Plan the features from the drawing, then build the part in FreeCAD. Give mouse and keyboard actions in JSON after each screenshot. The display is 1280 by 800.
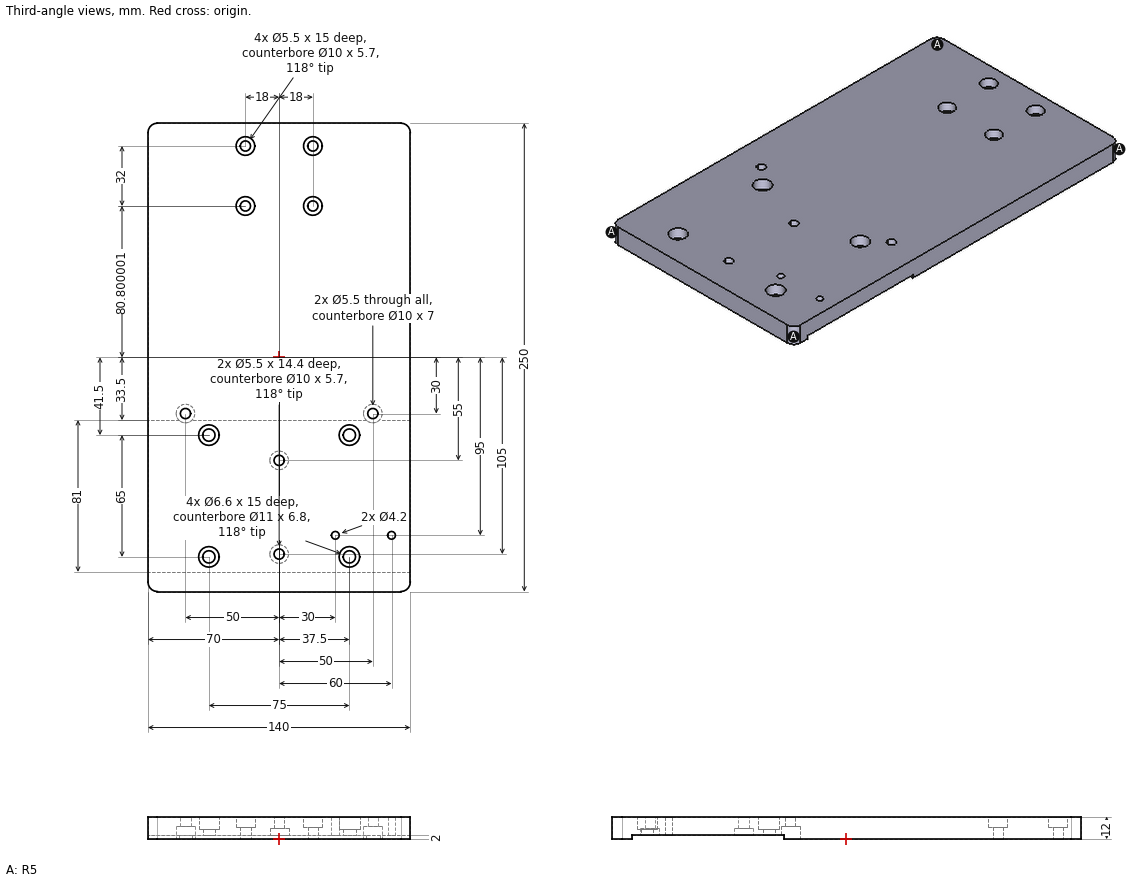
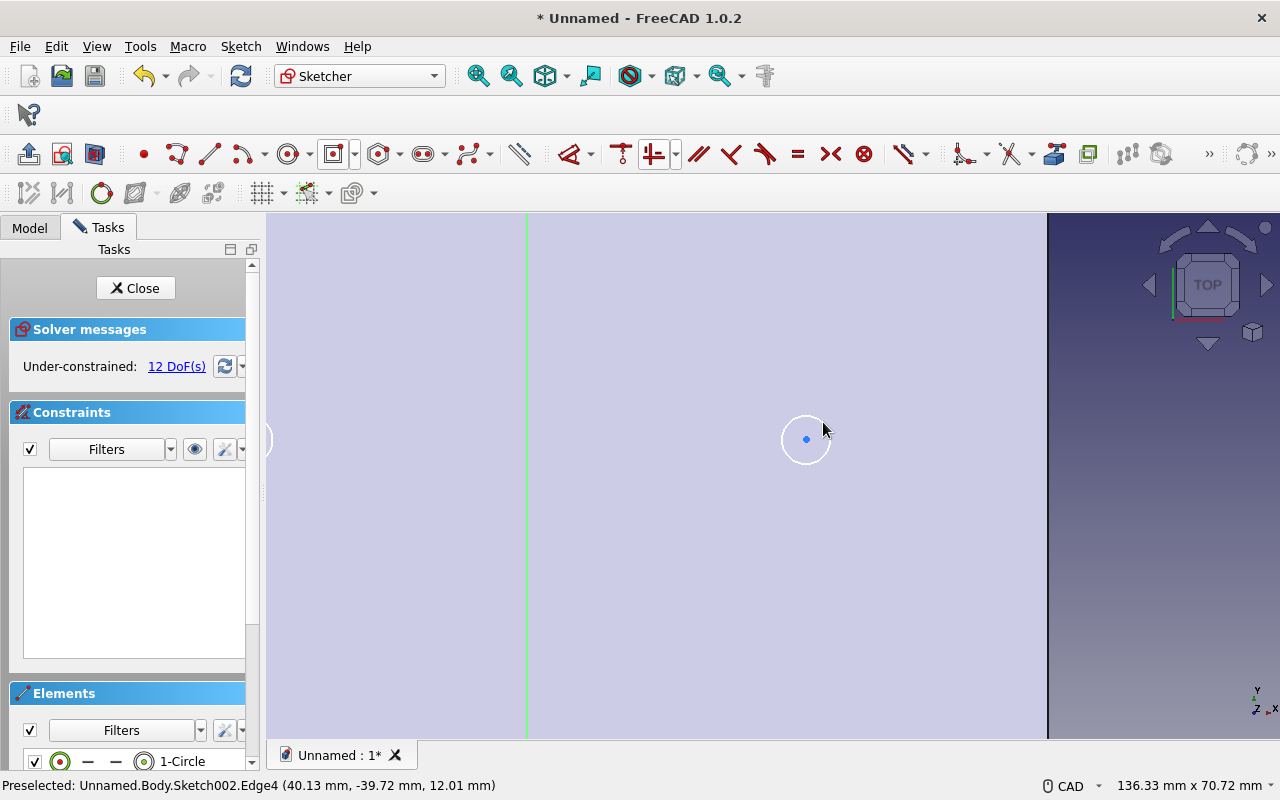
{"action": "scroll", "coordinate": [808, 439], "scroll_direction": "down", "scroll_amount": 5}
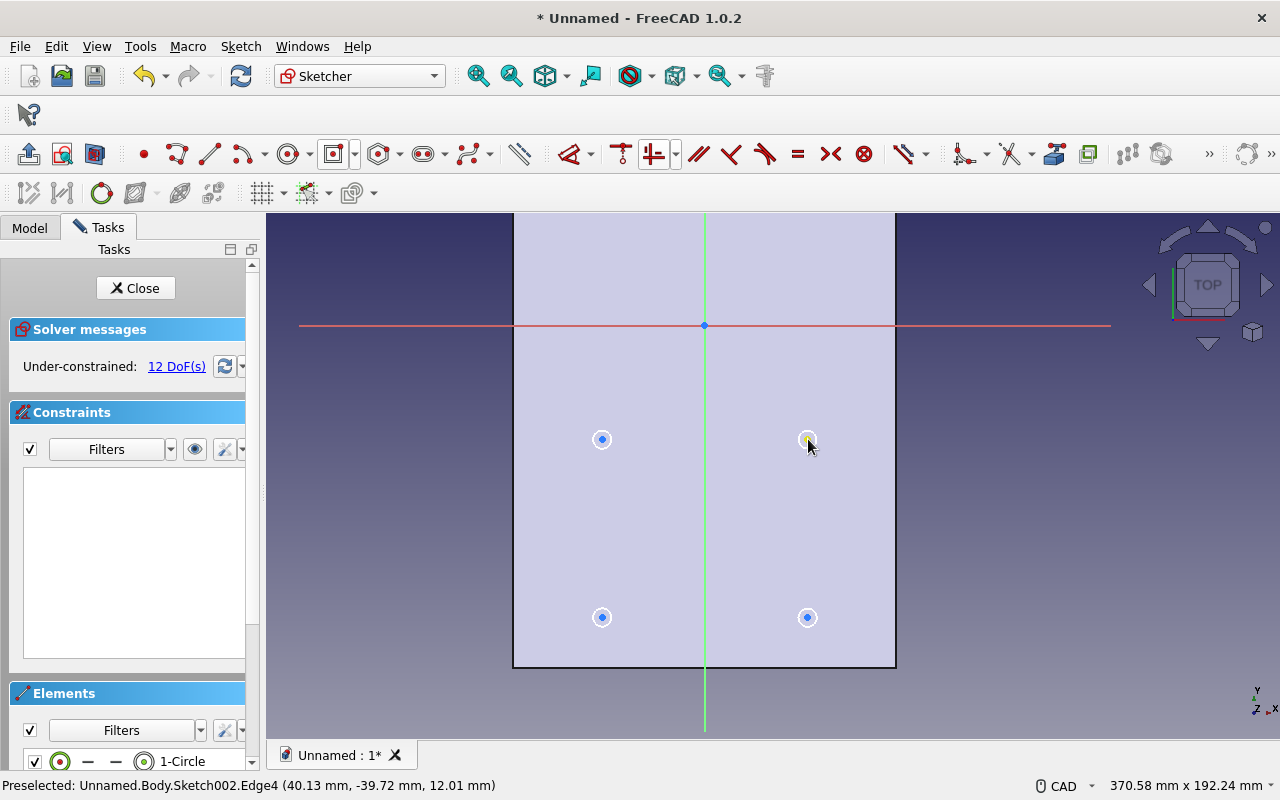
{"action": "scroll", "coordinate": [814, 611], "scroll_direction": "up", "scroll_amount": 3}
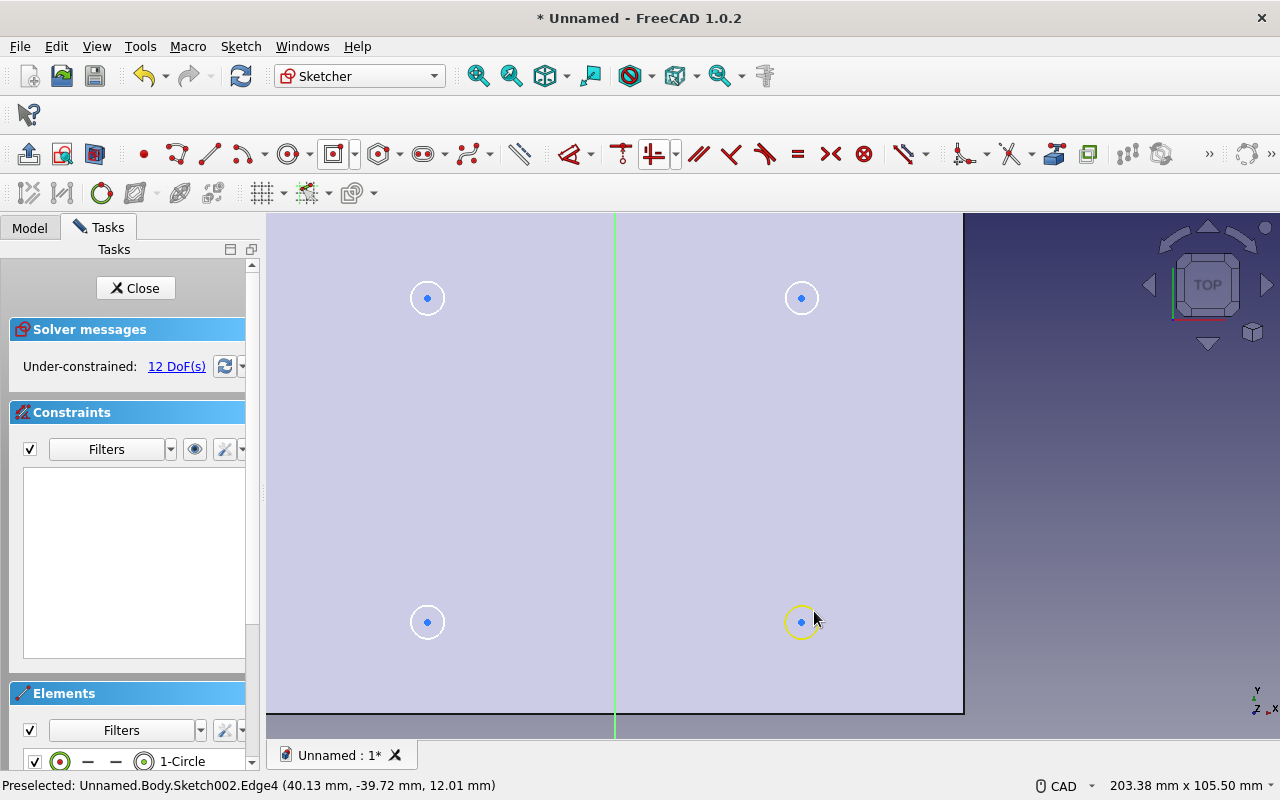
{"action": "left_click", "coordinate": [814, 611]}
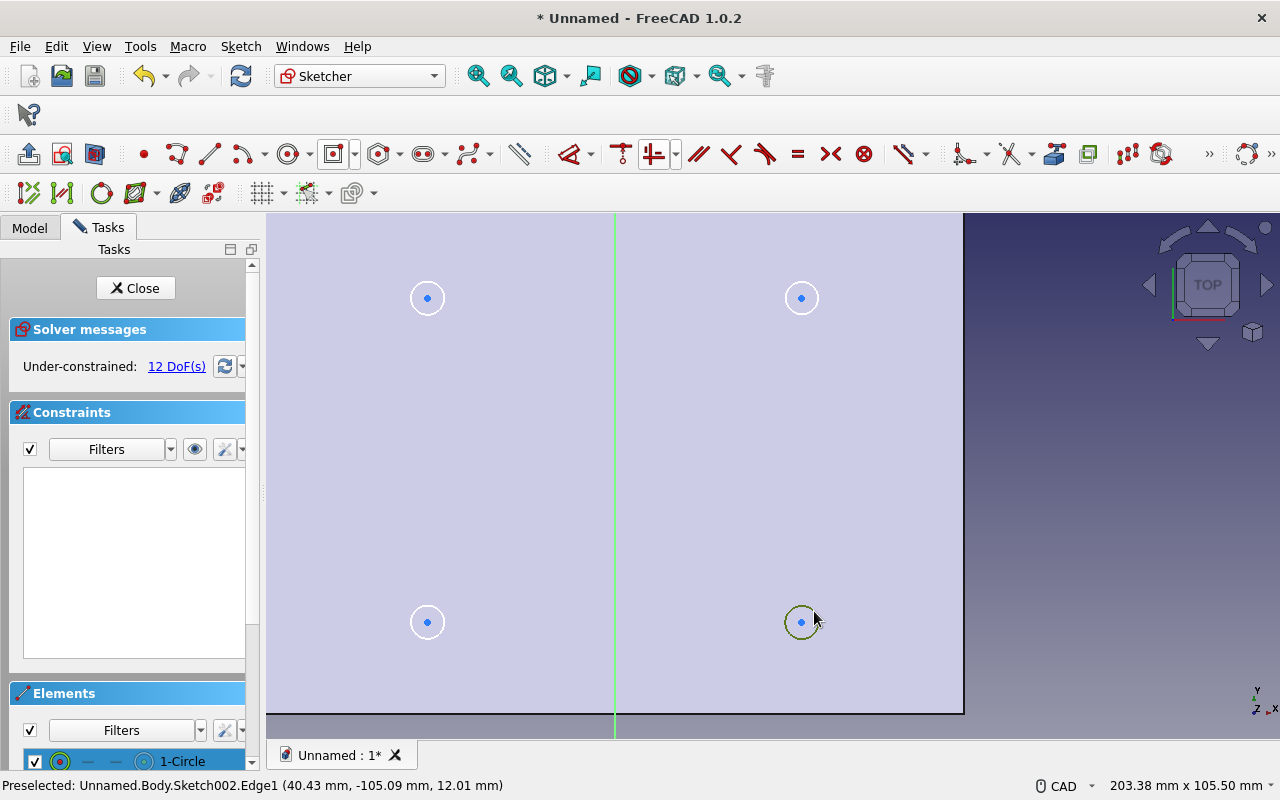
{"action": "left_click", "coordinate": [439, 610]}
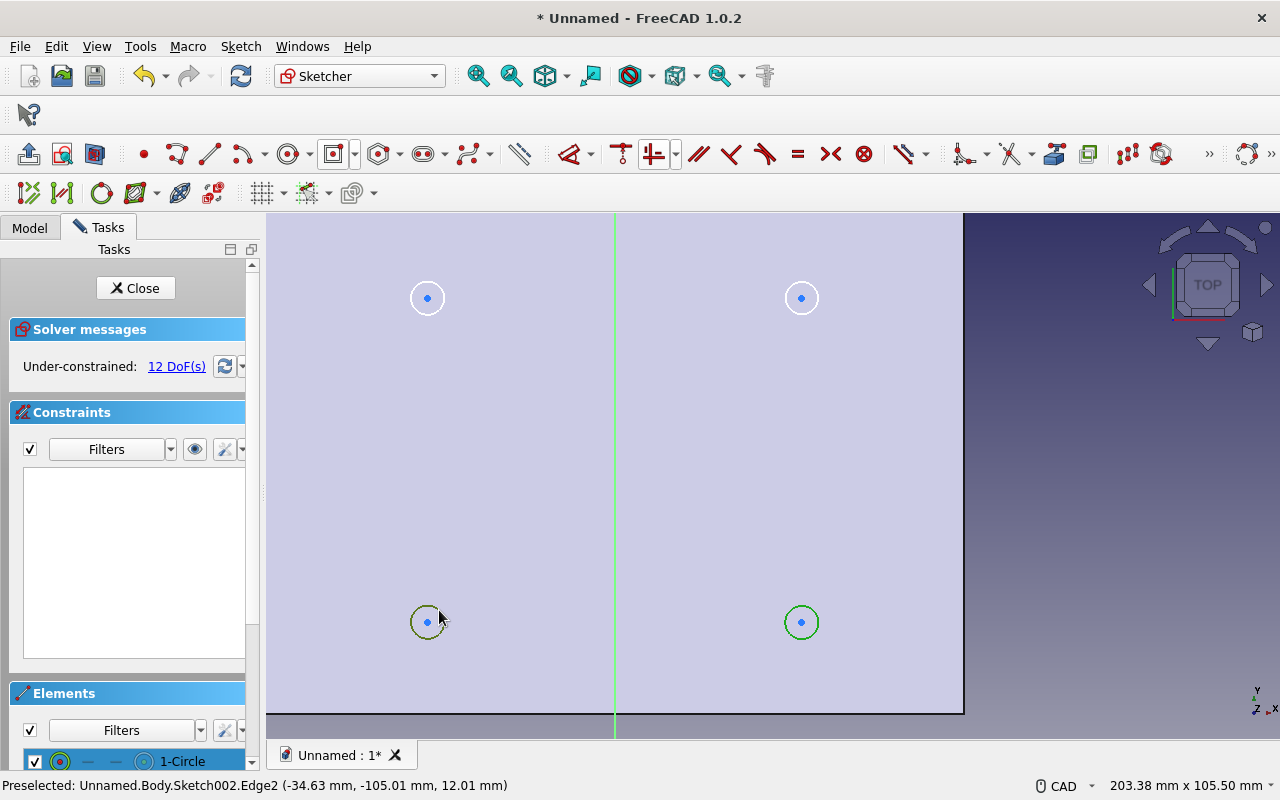
{"action": "left_click", "coordinate": [439, 286]}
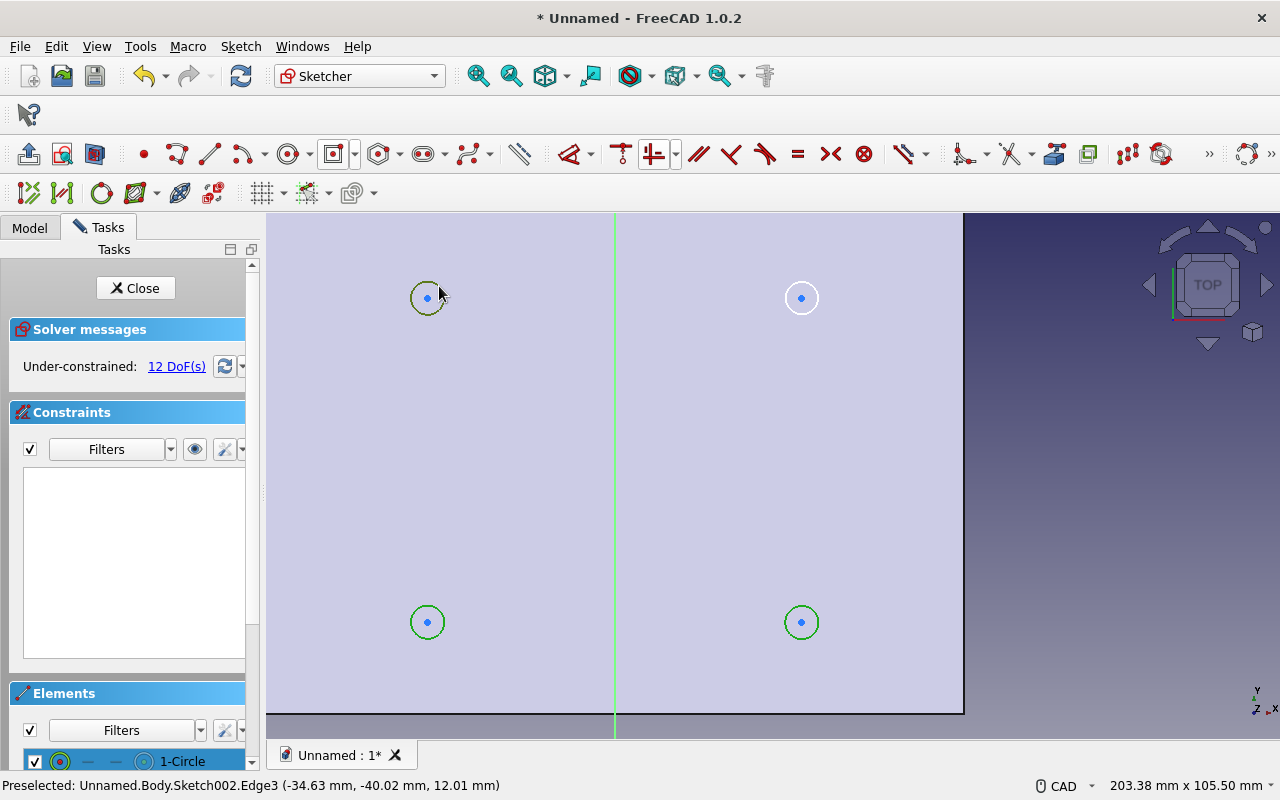
{"action": "left_click", "coordinate": [813, 287]}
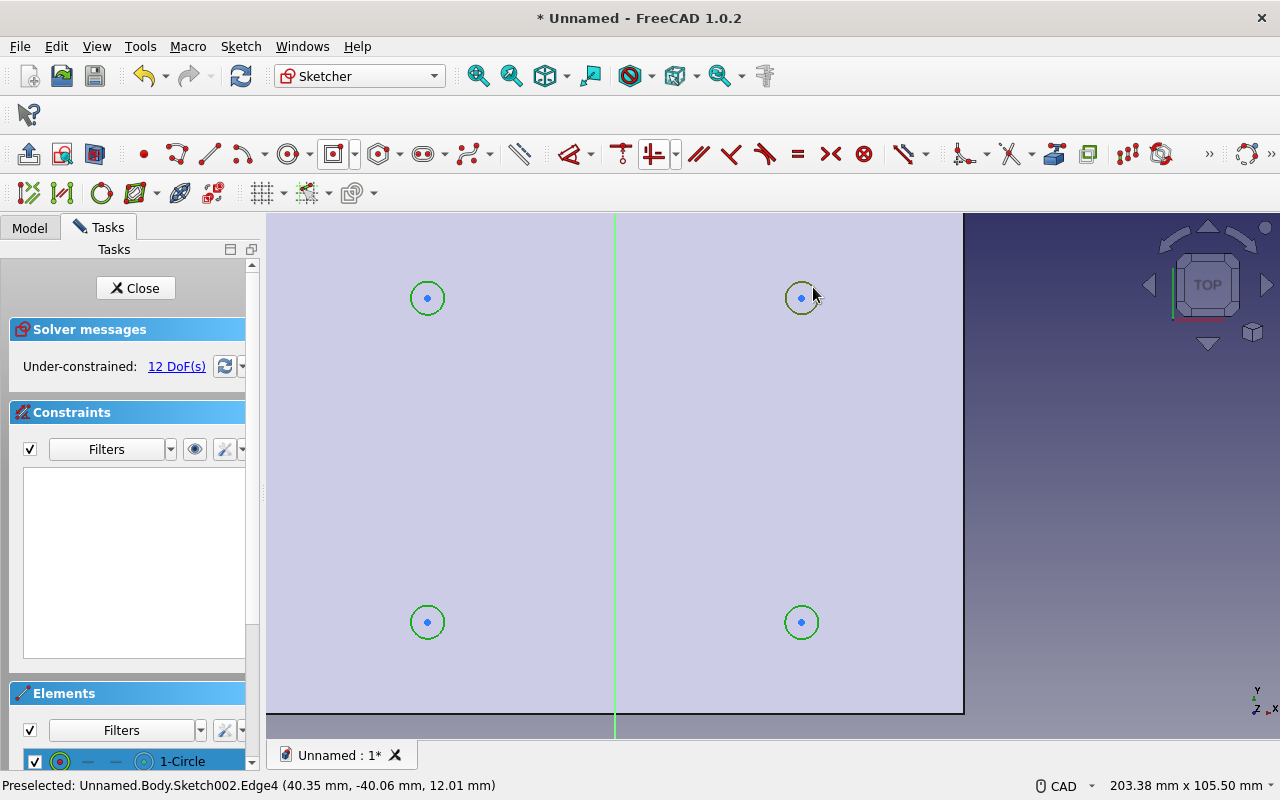
{"action": "left_click", "coordinate": [798, 154]}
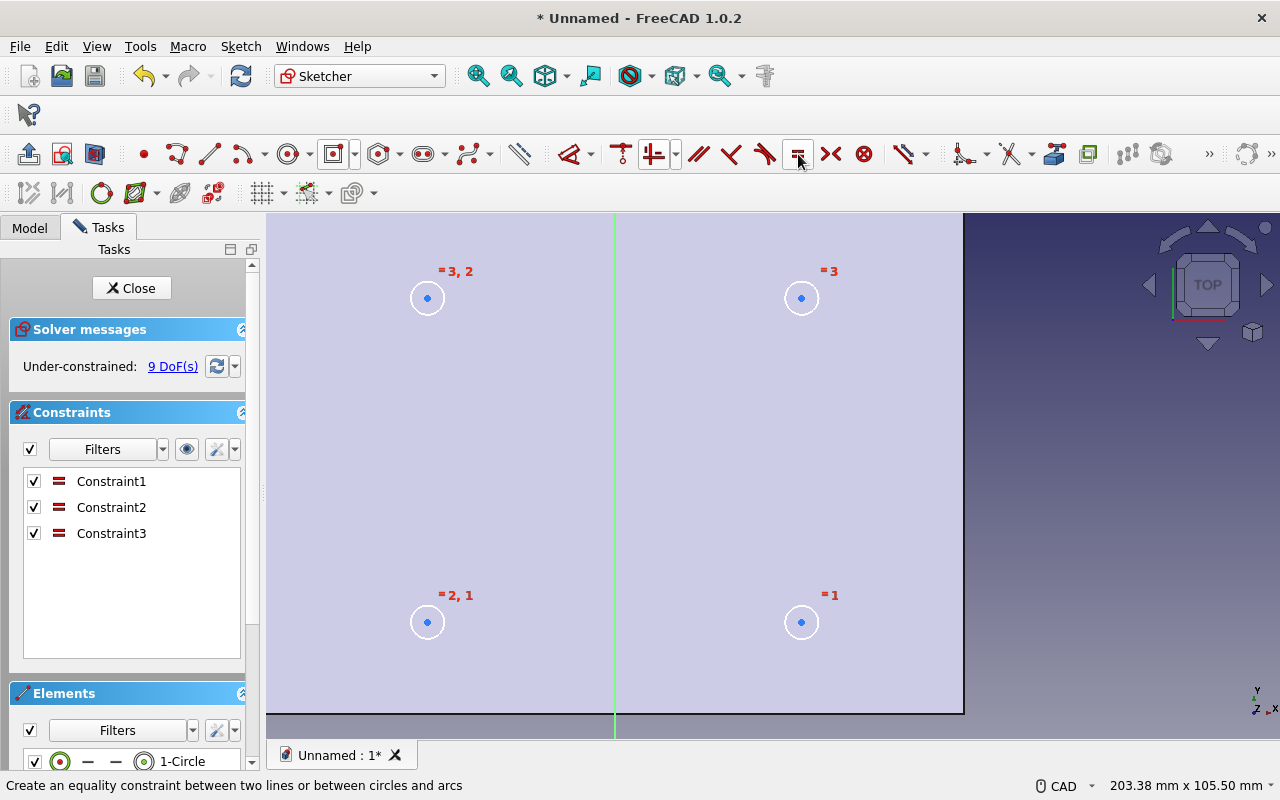
{"action": "left_click", "coordinate": [802, 623]}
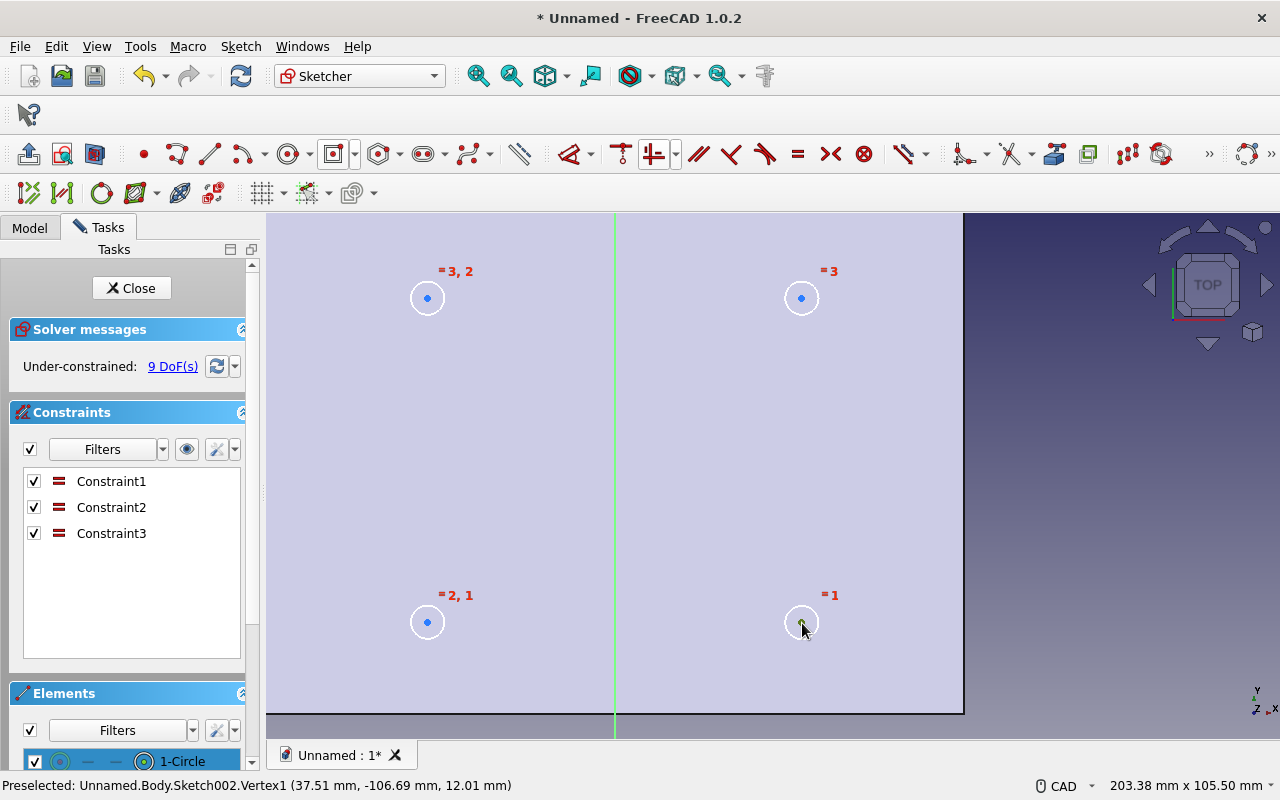
{"action": "left_click", "coordinate": [428, 622]}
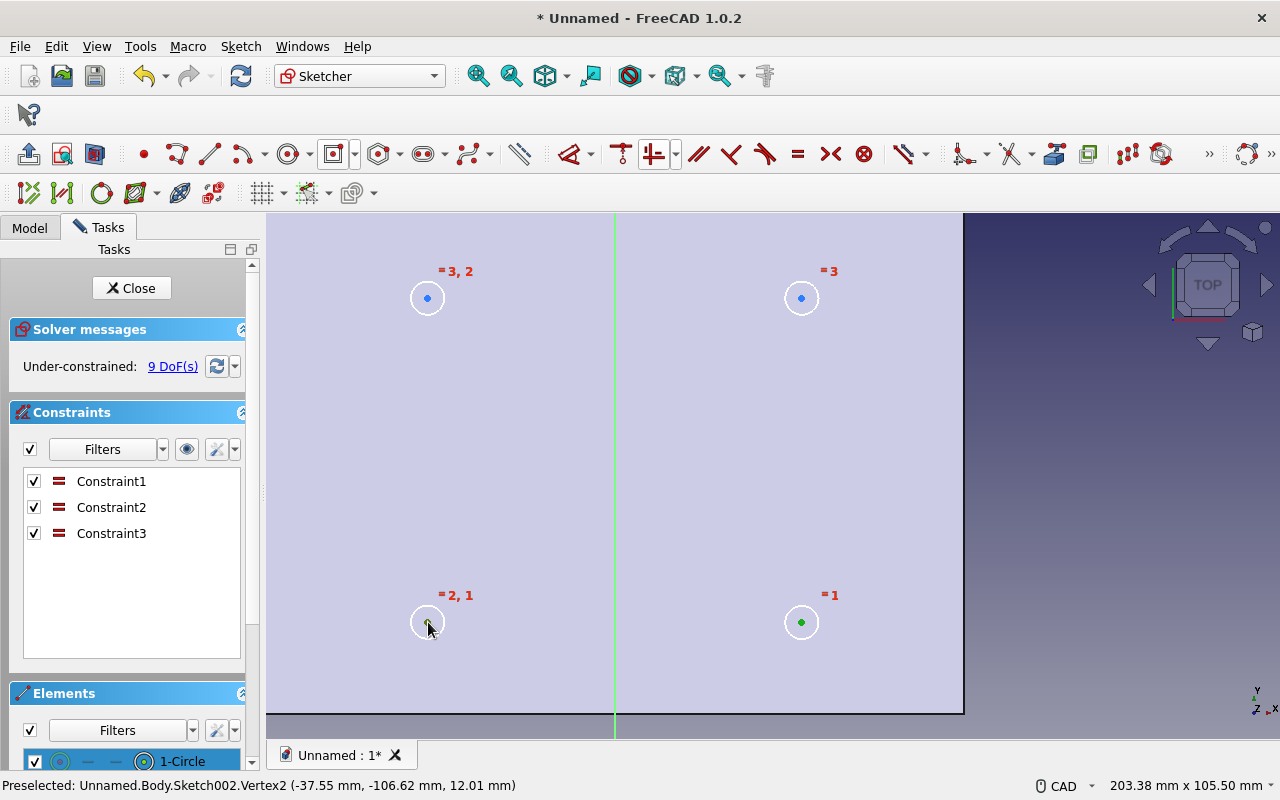
{"action": "left_click", "coordinate": [676, 154]}